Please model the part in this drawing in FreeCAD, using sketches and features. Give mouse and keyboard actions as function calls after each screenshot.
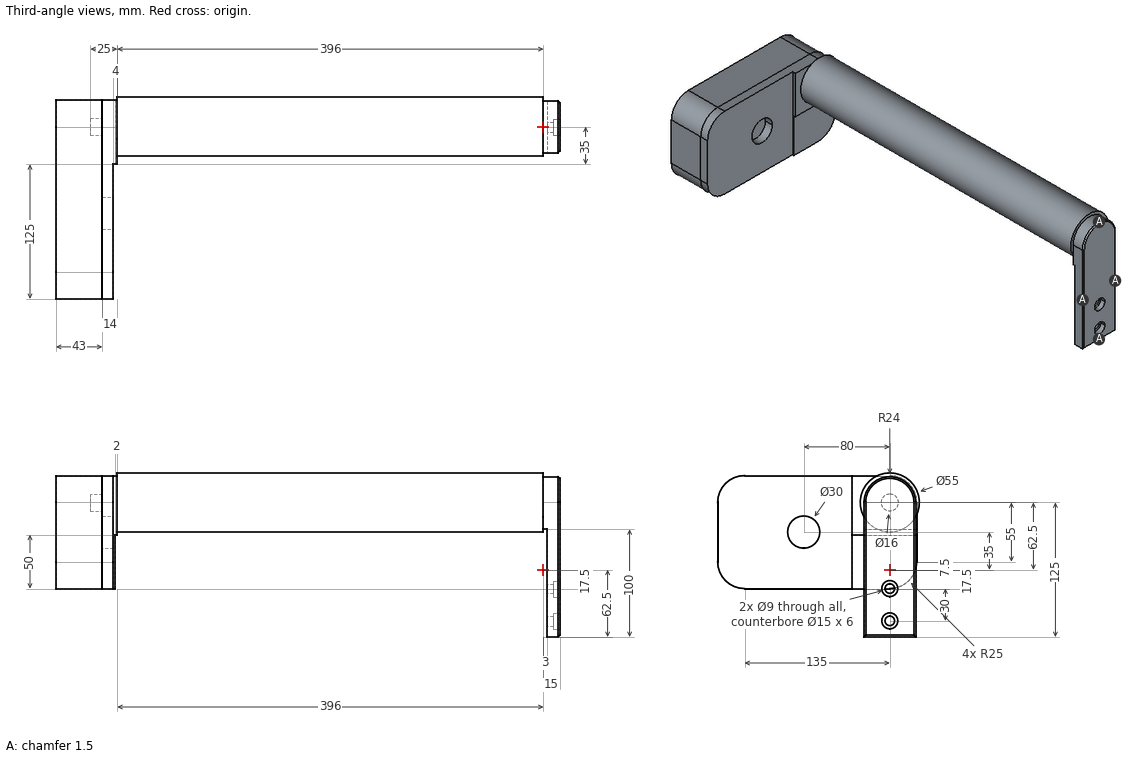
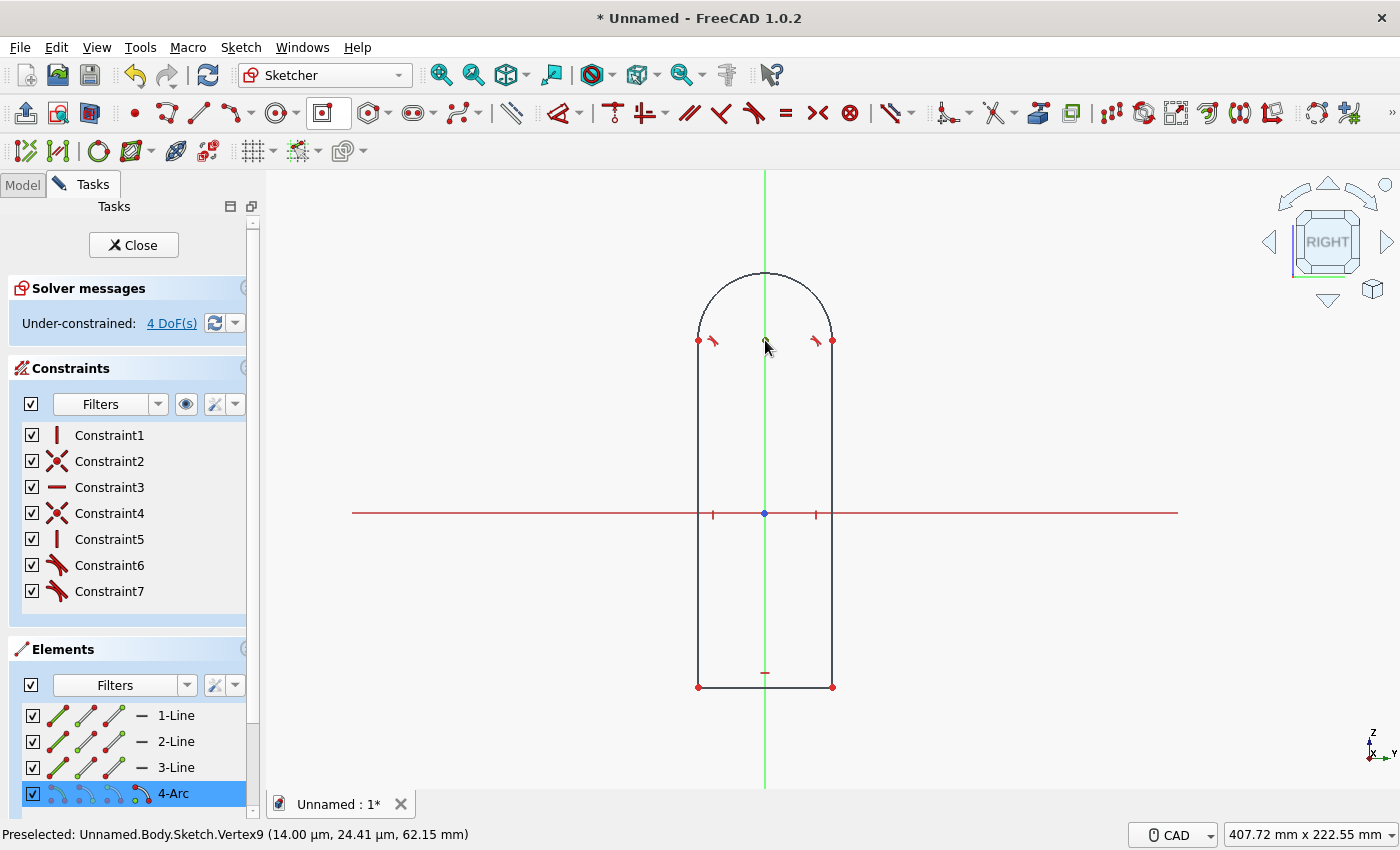
click(765, 721)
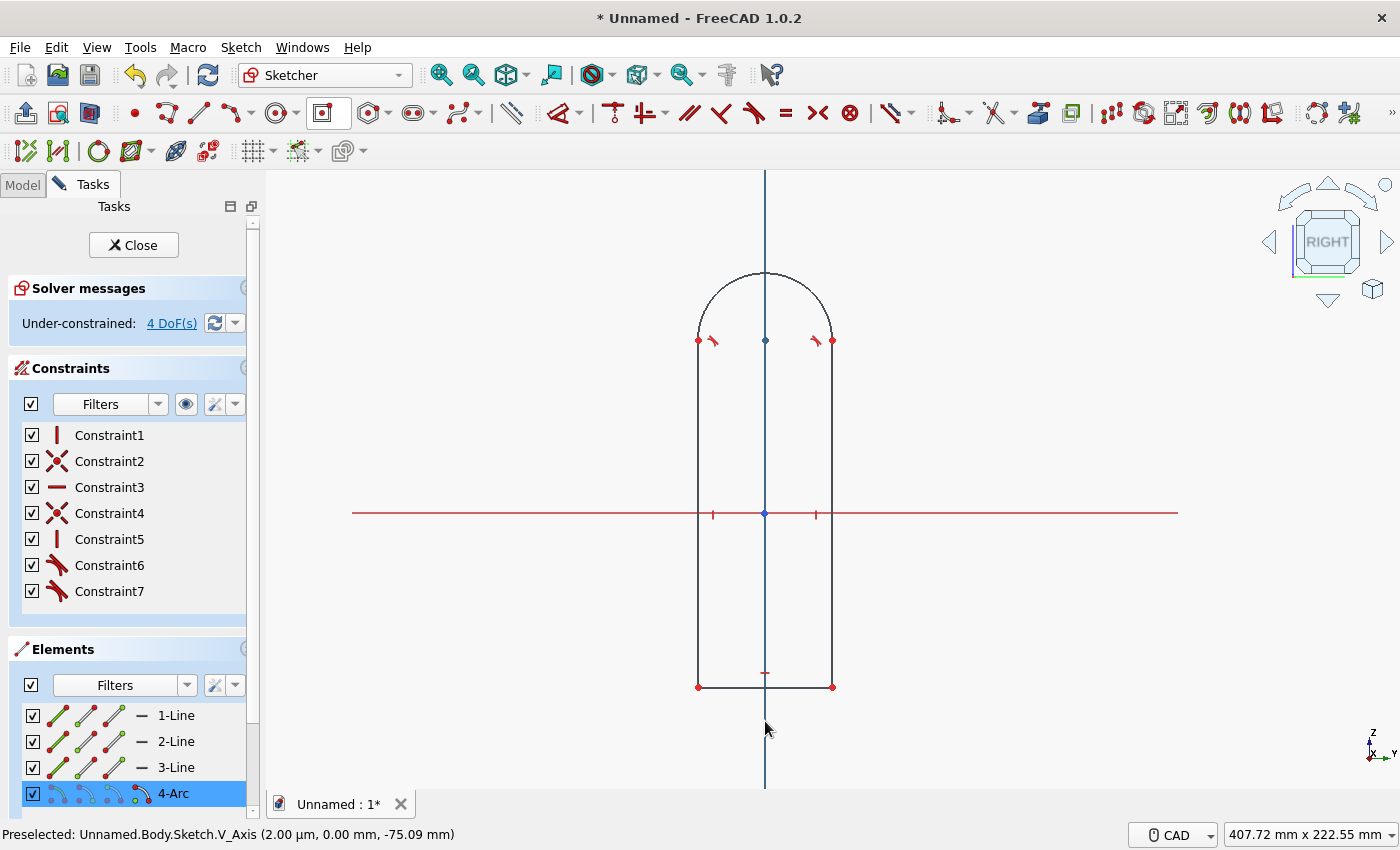
click(614, 114)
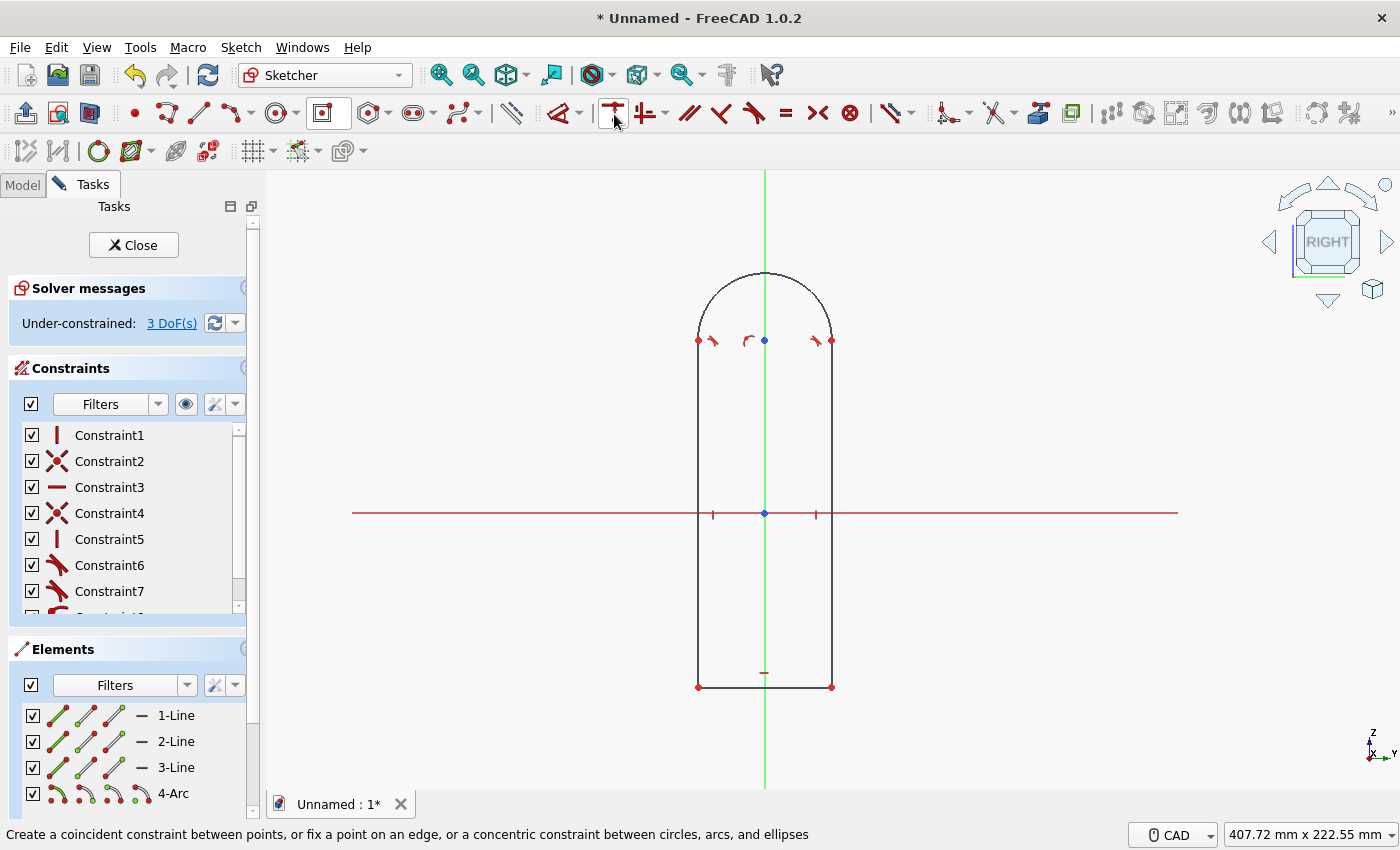
key(d)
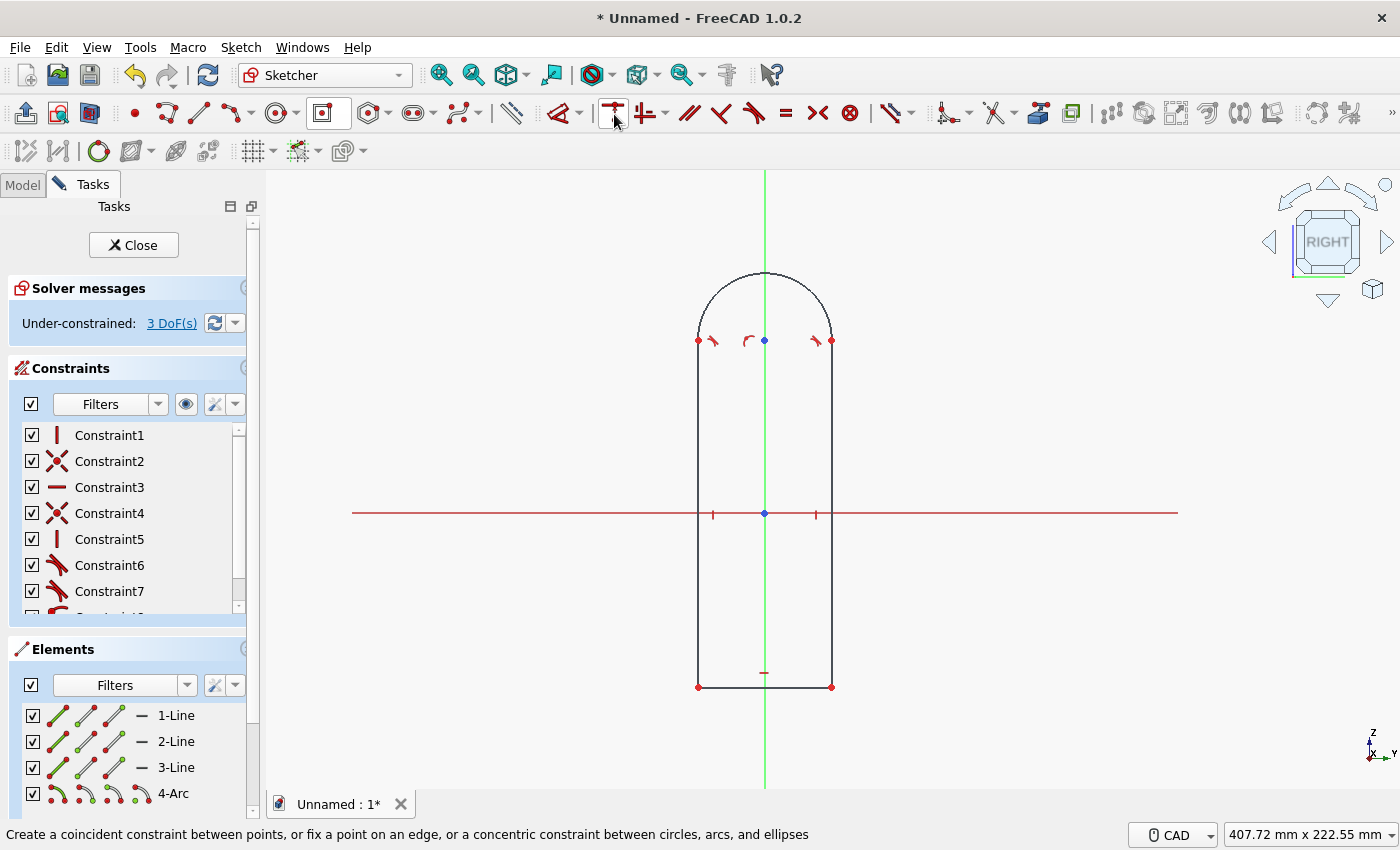
click(804, 286)
click(823, 260)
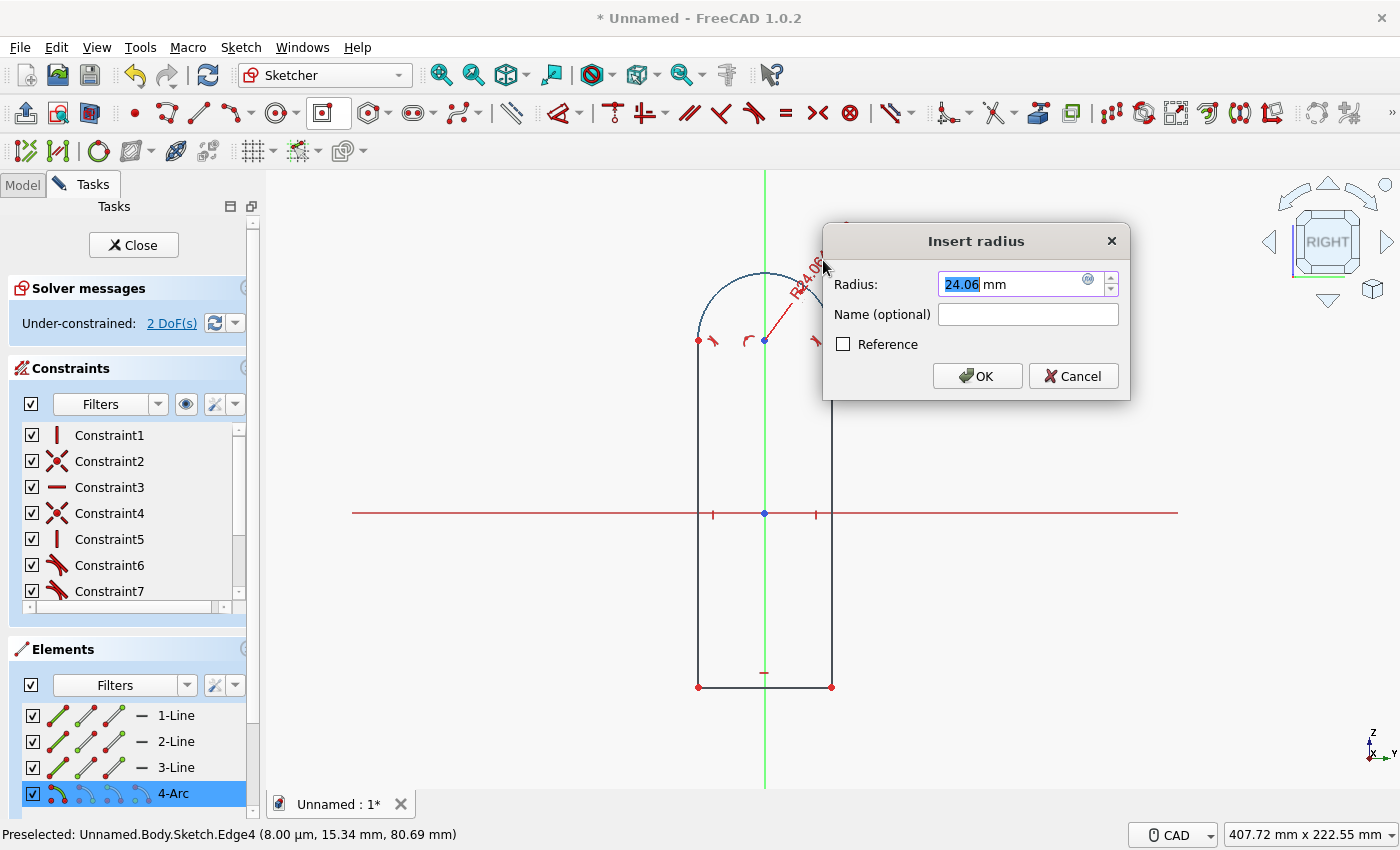
text(24)
key(Return)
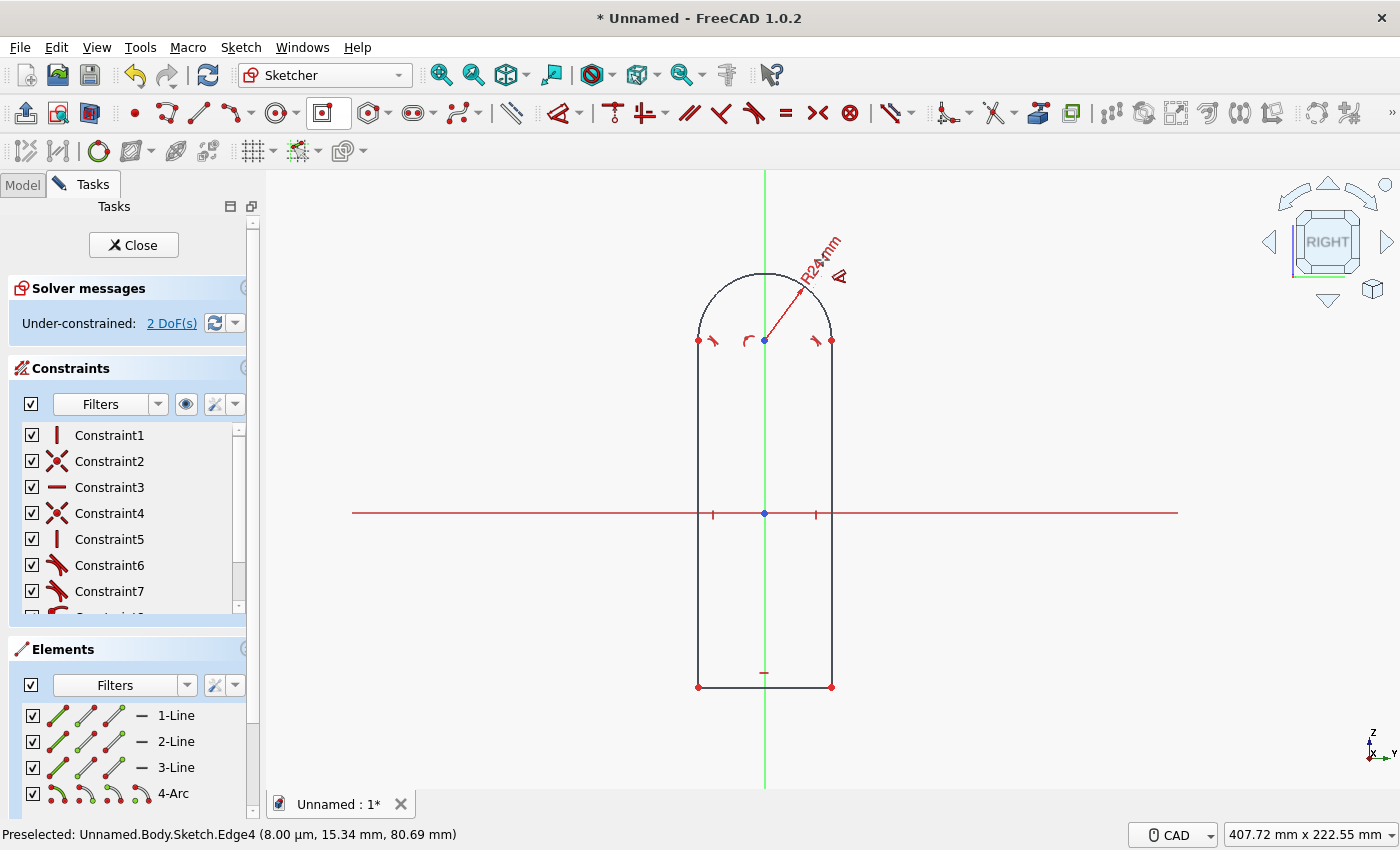
click(698, 445)
click(664, 434)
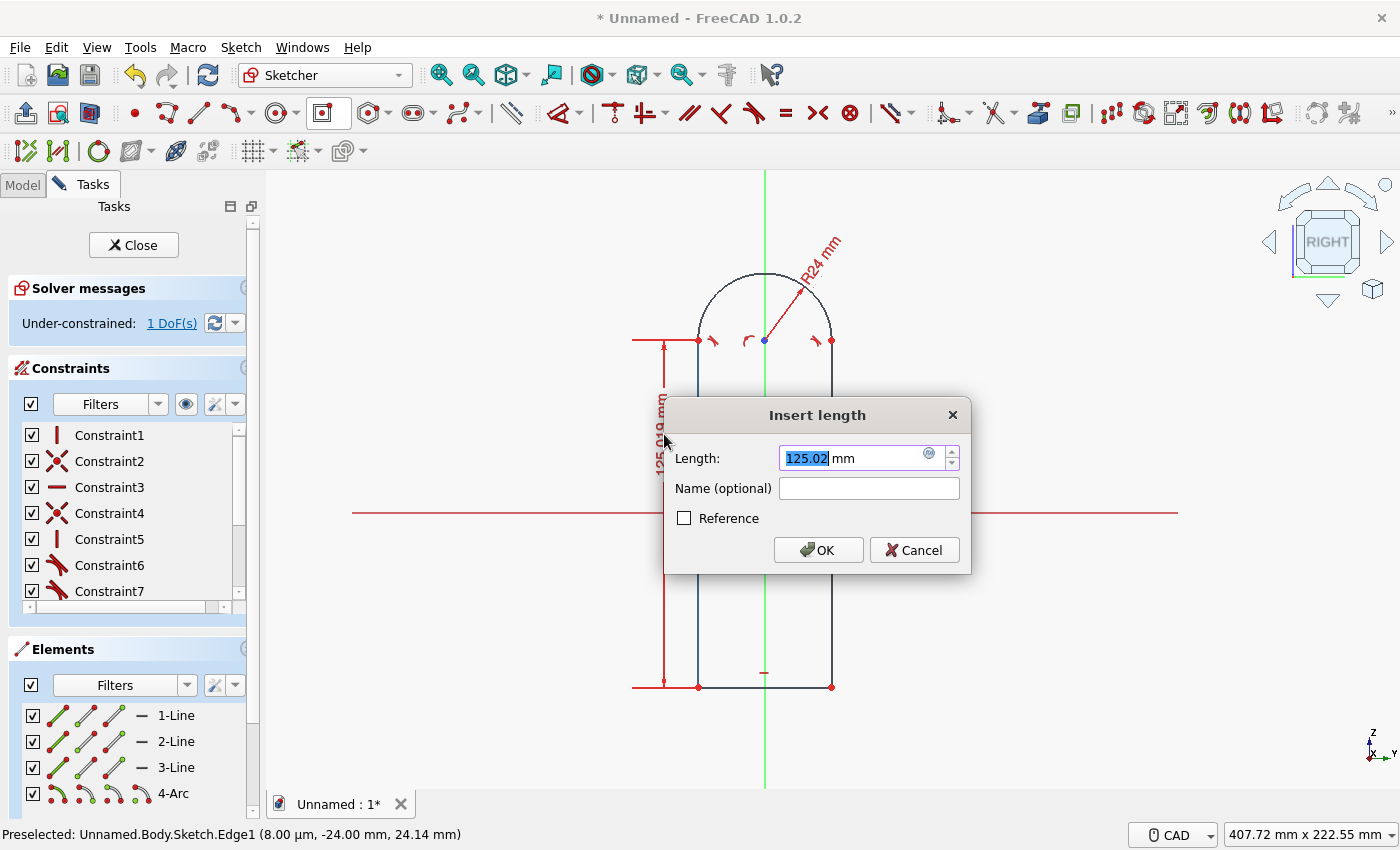
text(125)
key(Return)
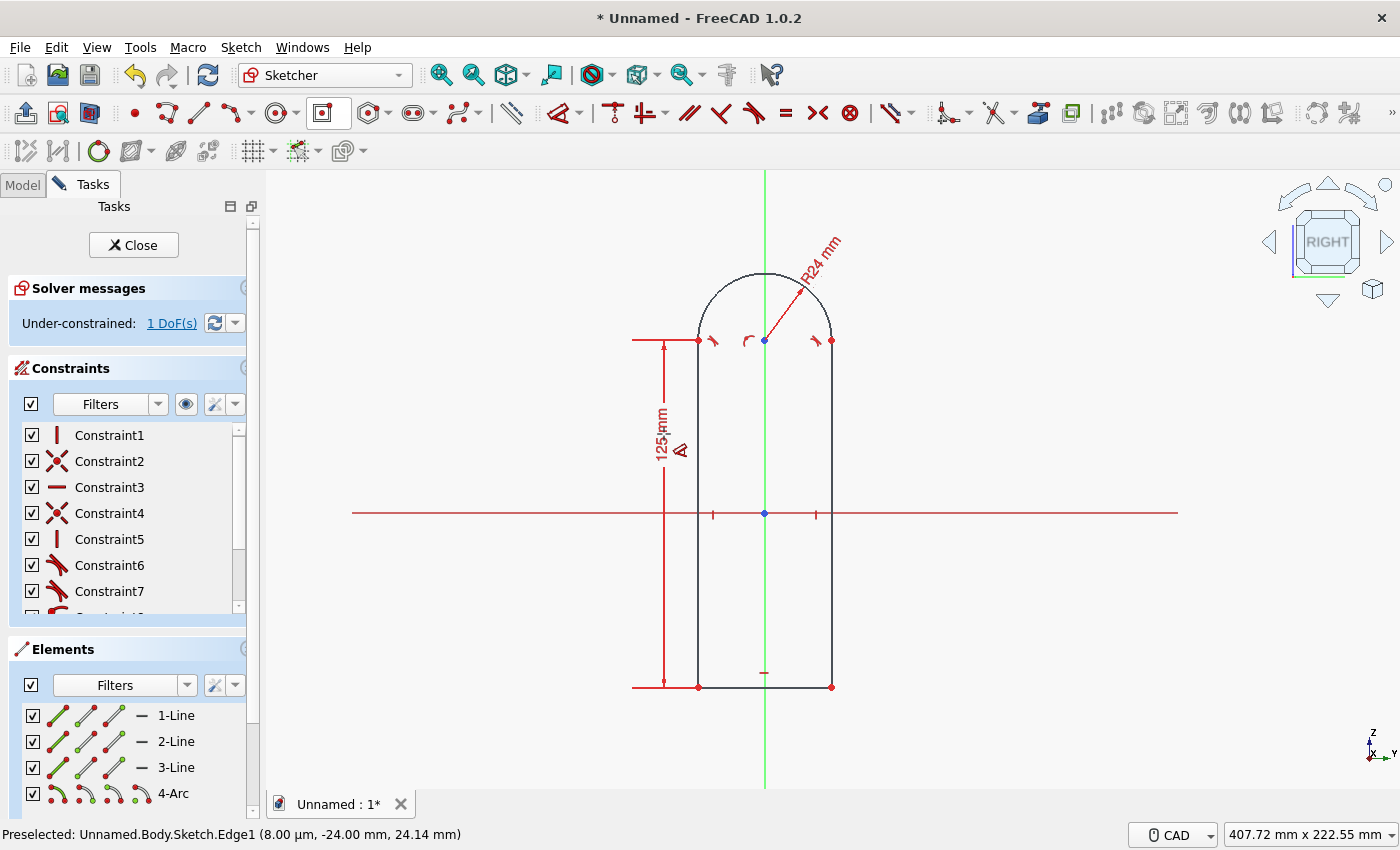
click(698, 340)
click(664, 387)